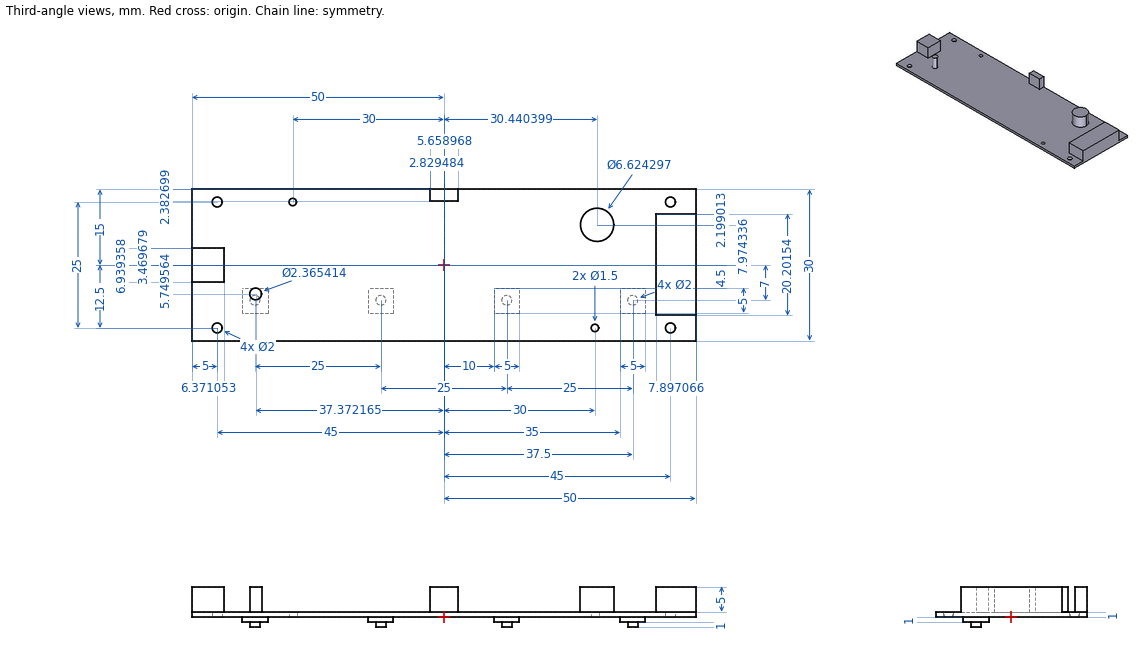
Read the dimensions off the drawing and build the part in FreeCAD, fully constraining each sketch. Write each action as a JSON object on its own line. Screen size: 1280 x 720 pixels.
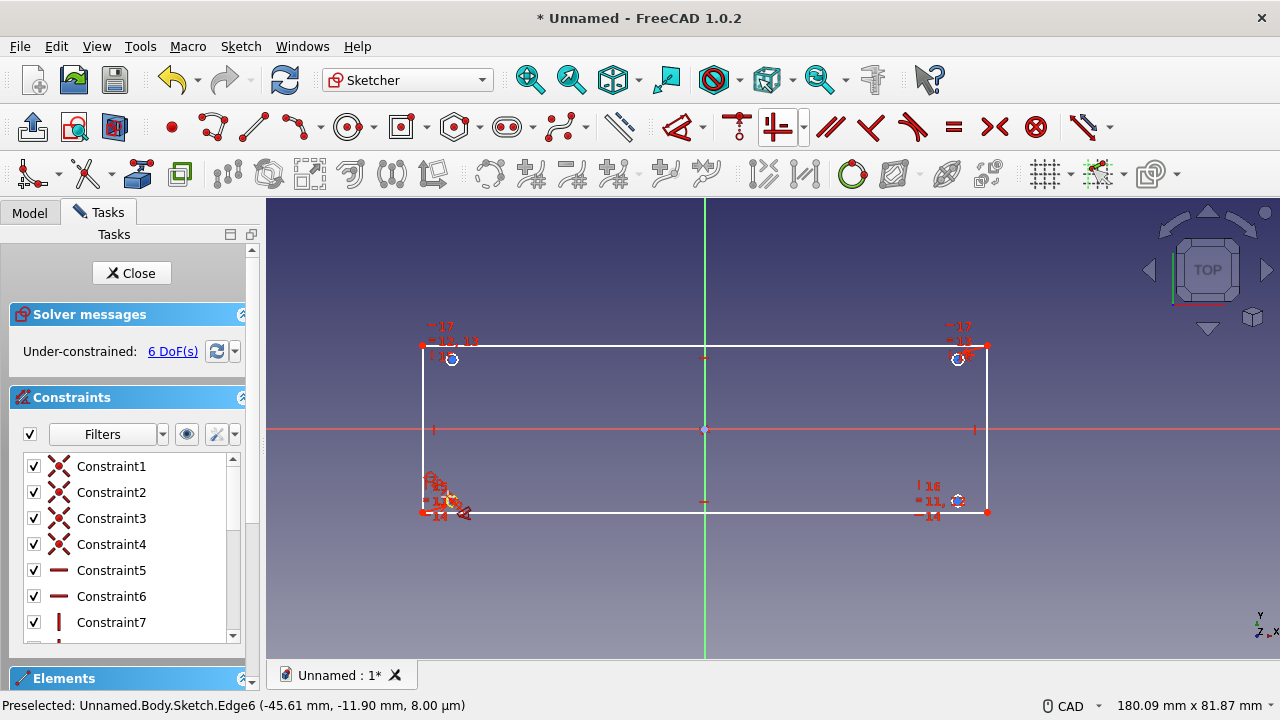
{"action": "left_click", "coordinate": [987, 463]}
{"action": "left_click", "coordinate": [1021, 391]}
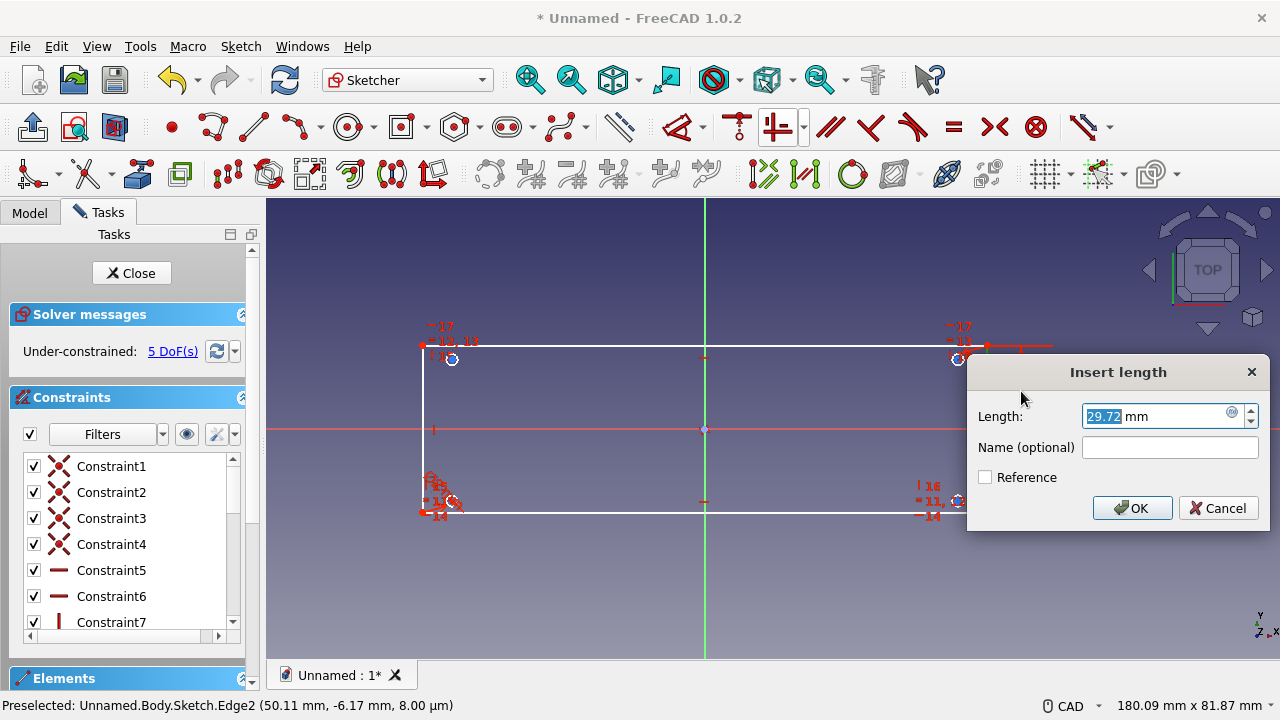
{"action": "type", "text": "30"}
{"action": "key", "text": "Return"}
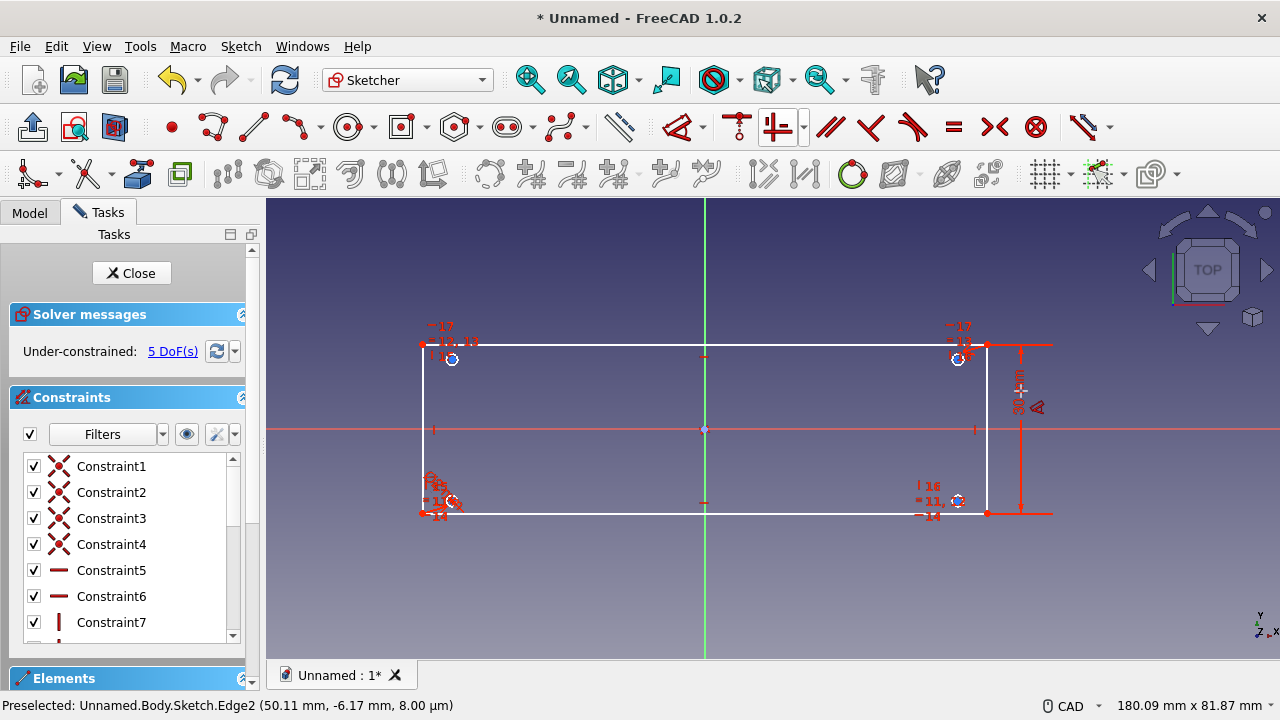
{"action": "left_click", "coordinate": [452, 501]}
{"action": "left_click", "coordinate": [578, 535]}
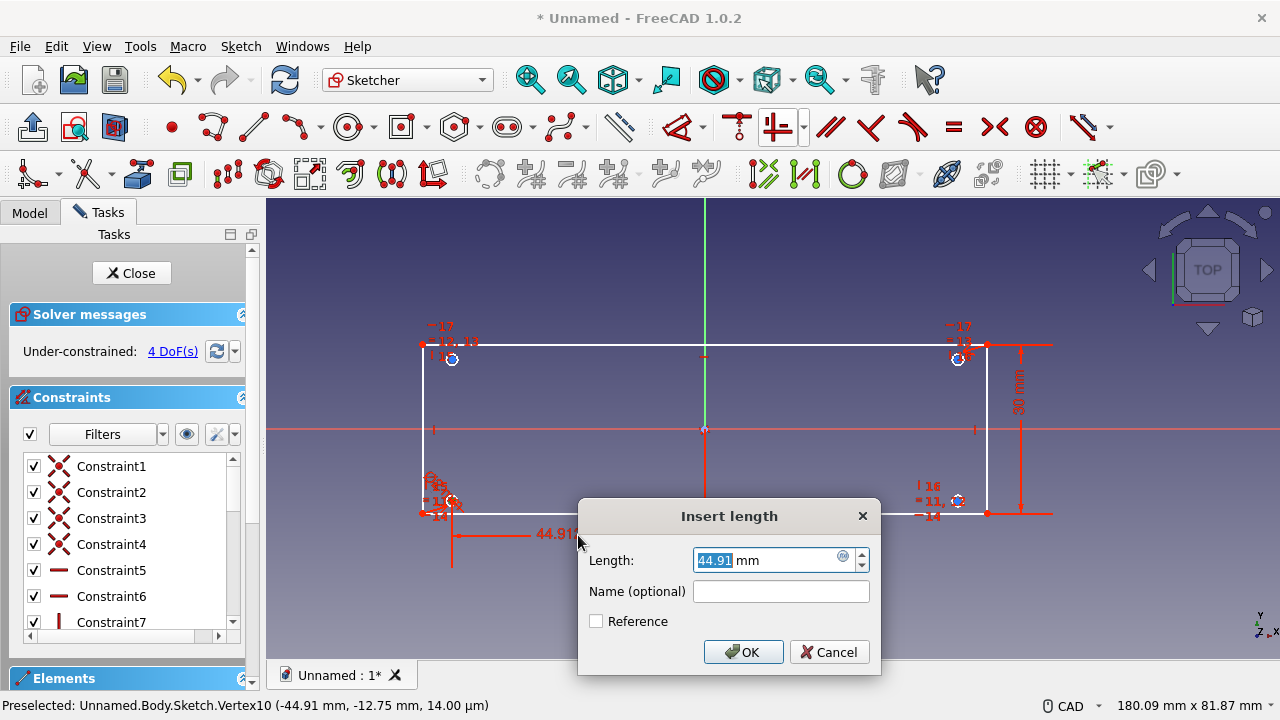
{"action": "type", "text": "45"}
{"action": "key", "text": "Return"}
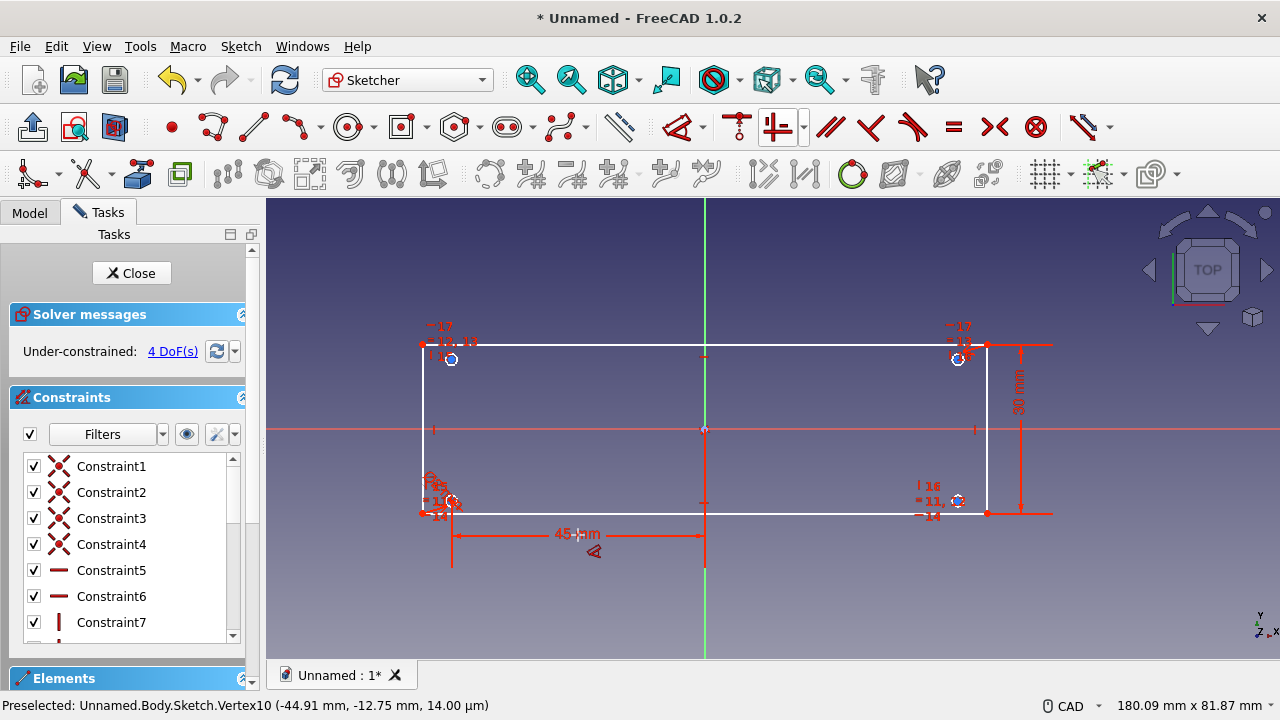
{"action": "left_click", "coordinate": [958, 501]}
{"action": "left_click", "coordinate": [831, 535]}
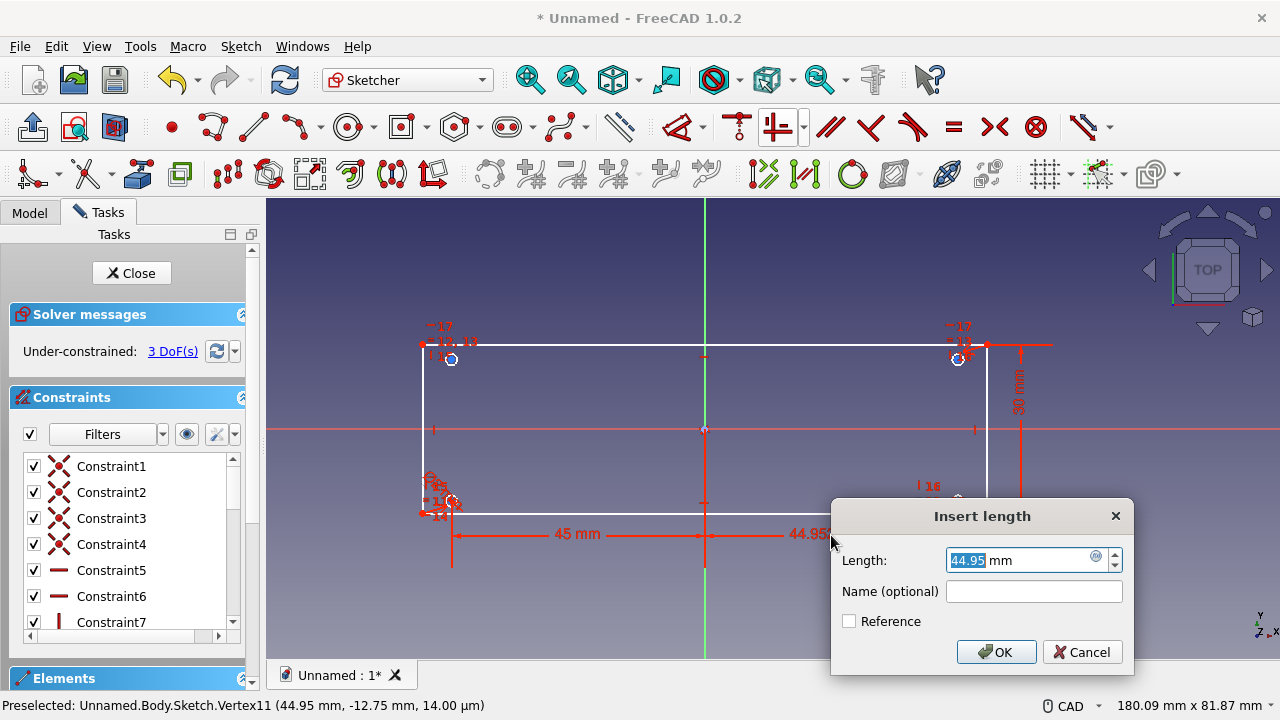
{"action": "type", "text": "45"}
{"action": "key", "text": "Return"}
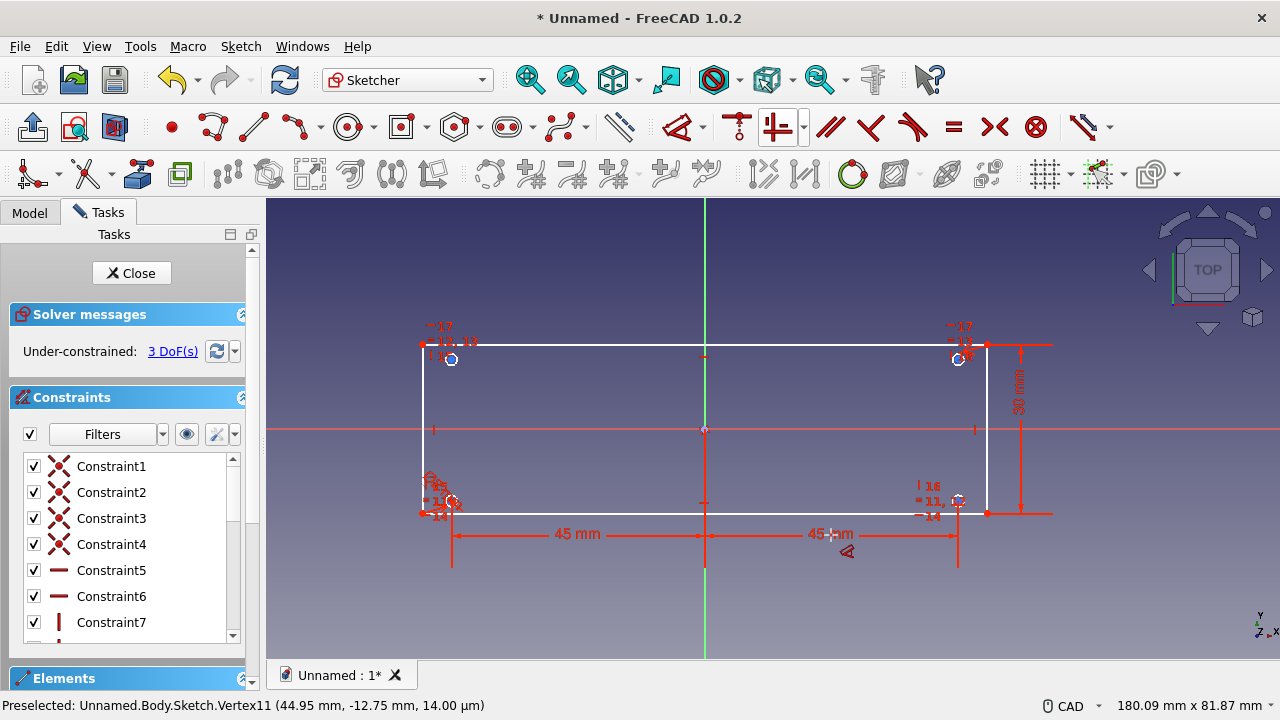
{"action": "scroll", "coordinate": [423, 514], "scroll_direction": "up", "scroll_amount": 2}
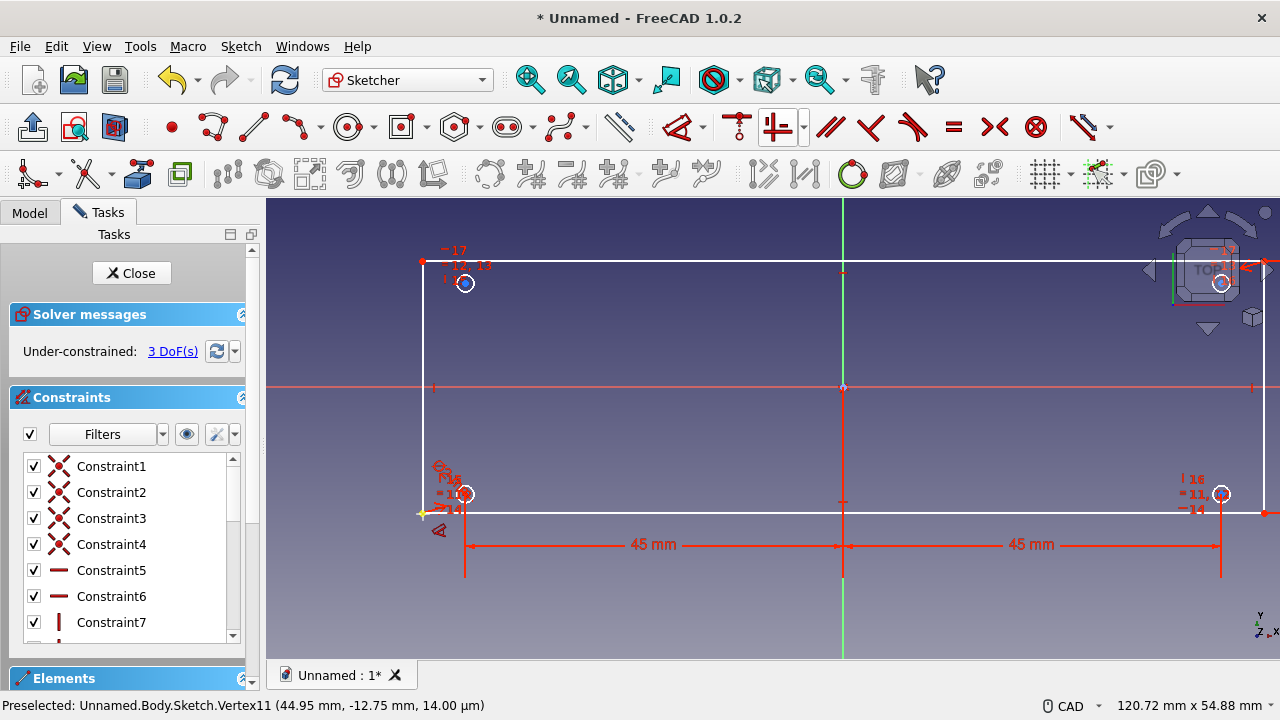
{"action": "left_click", "coordinate": [423, 513]}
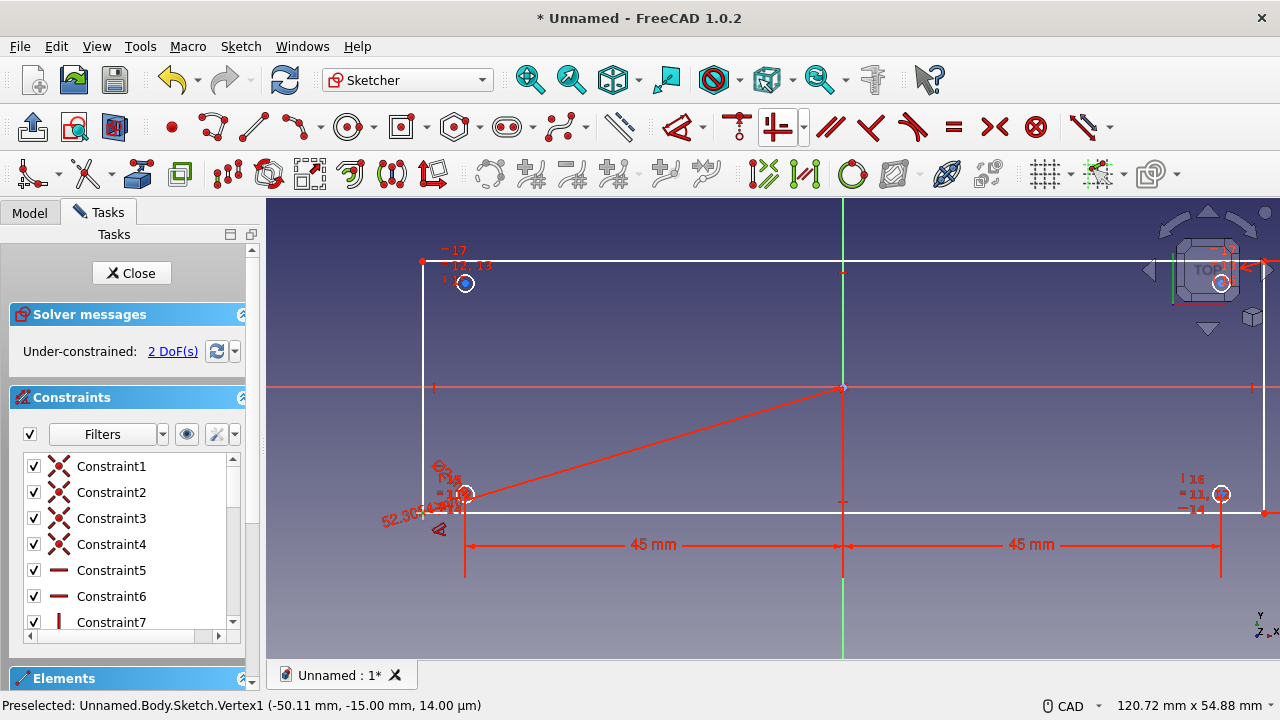
{"action": "left_click", "coordinate": [465, 494]}
{"action": "left_click", "coordinate": [444, 547]}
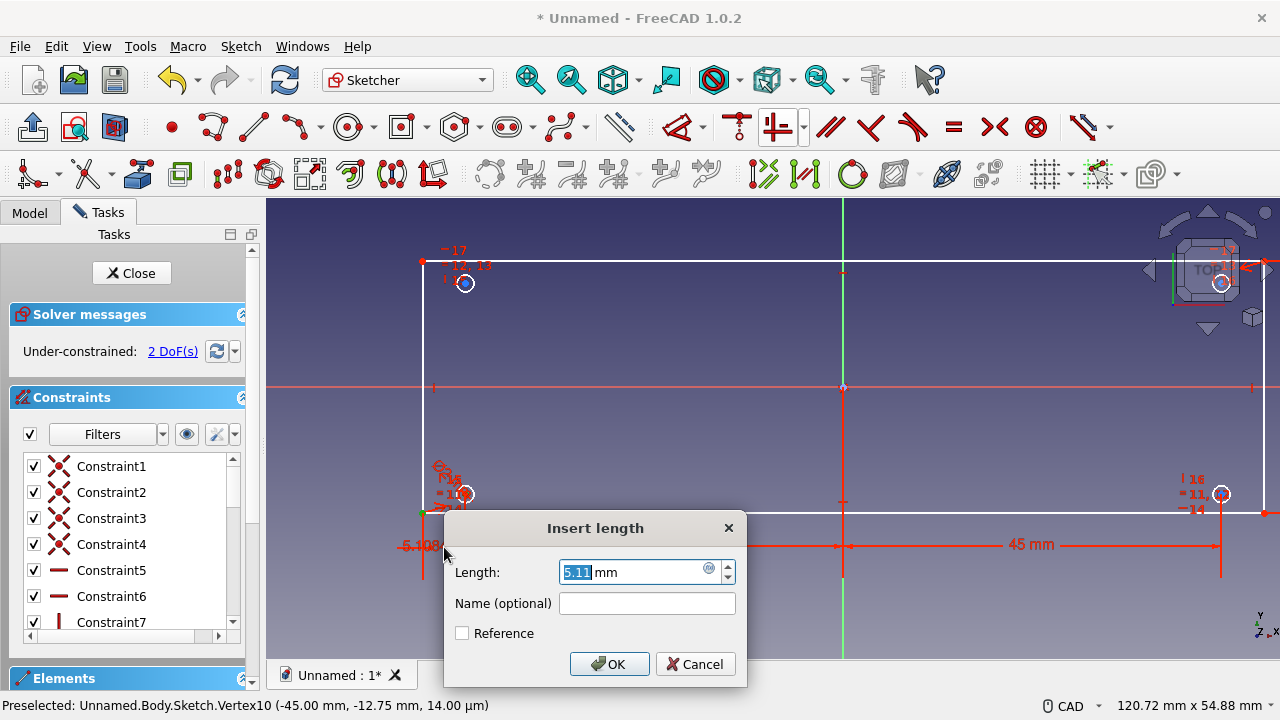
{"action": "type", "text": "5"}
{"action": "key", "text": "Return"}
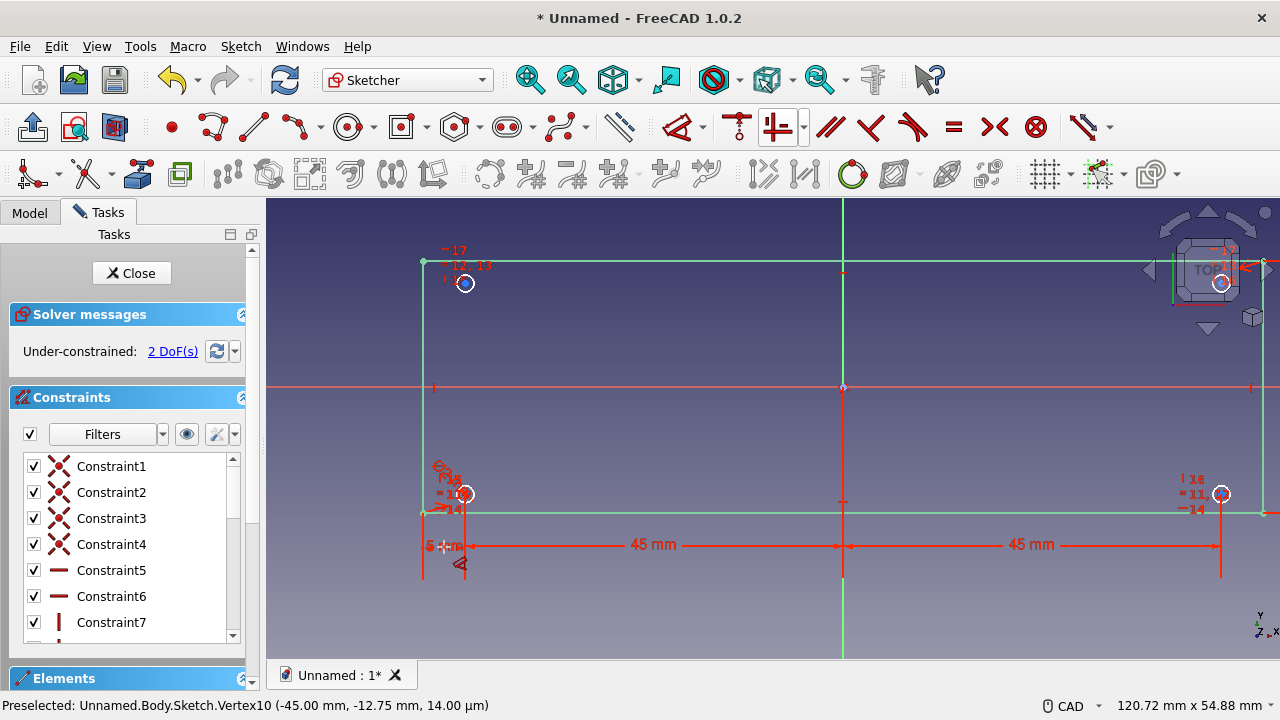
{"action": "left_click", "coordinate": [465, 494]}